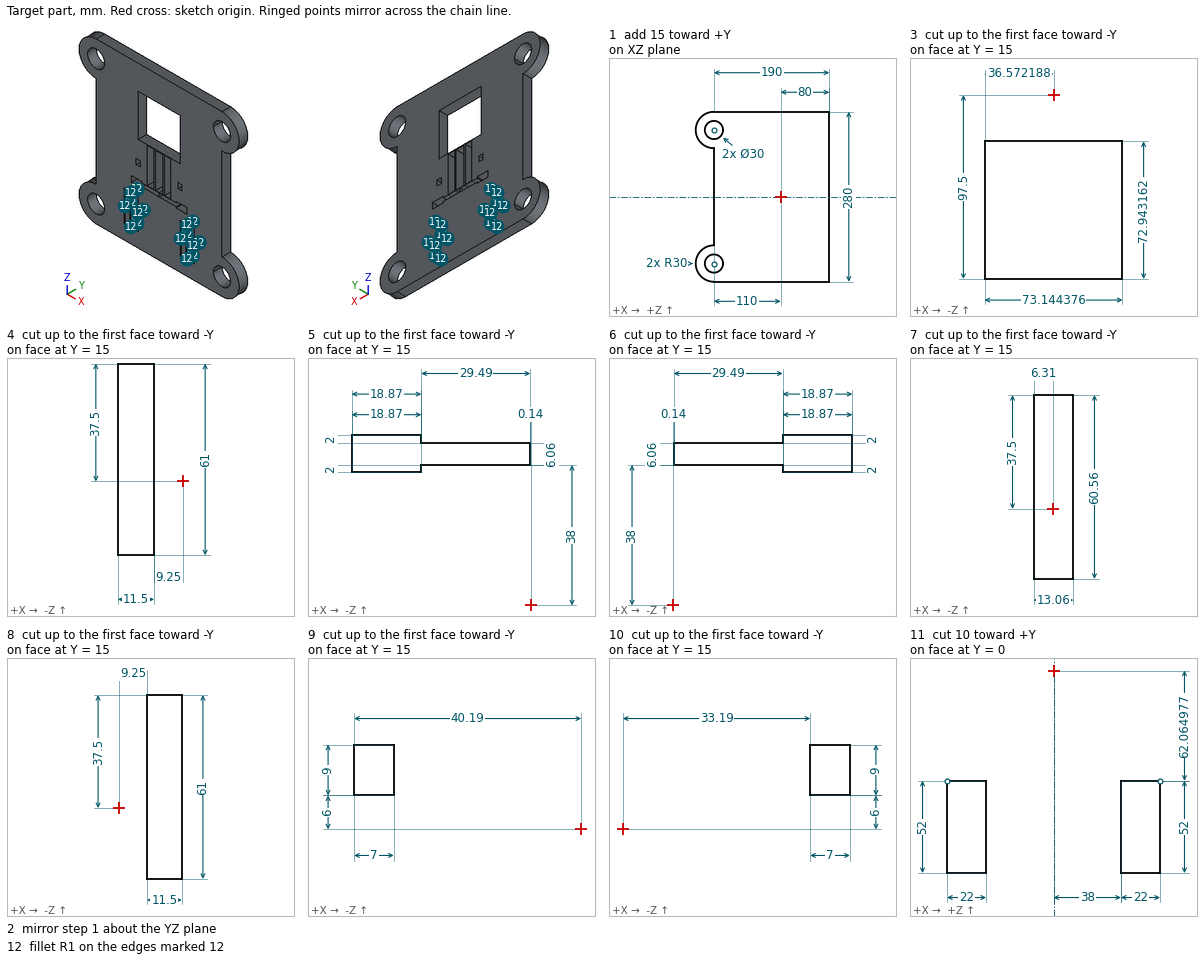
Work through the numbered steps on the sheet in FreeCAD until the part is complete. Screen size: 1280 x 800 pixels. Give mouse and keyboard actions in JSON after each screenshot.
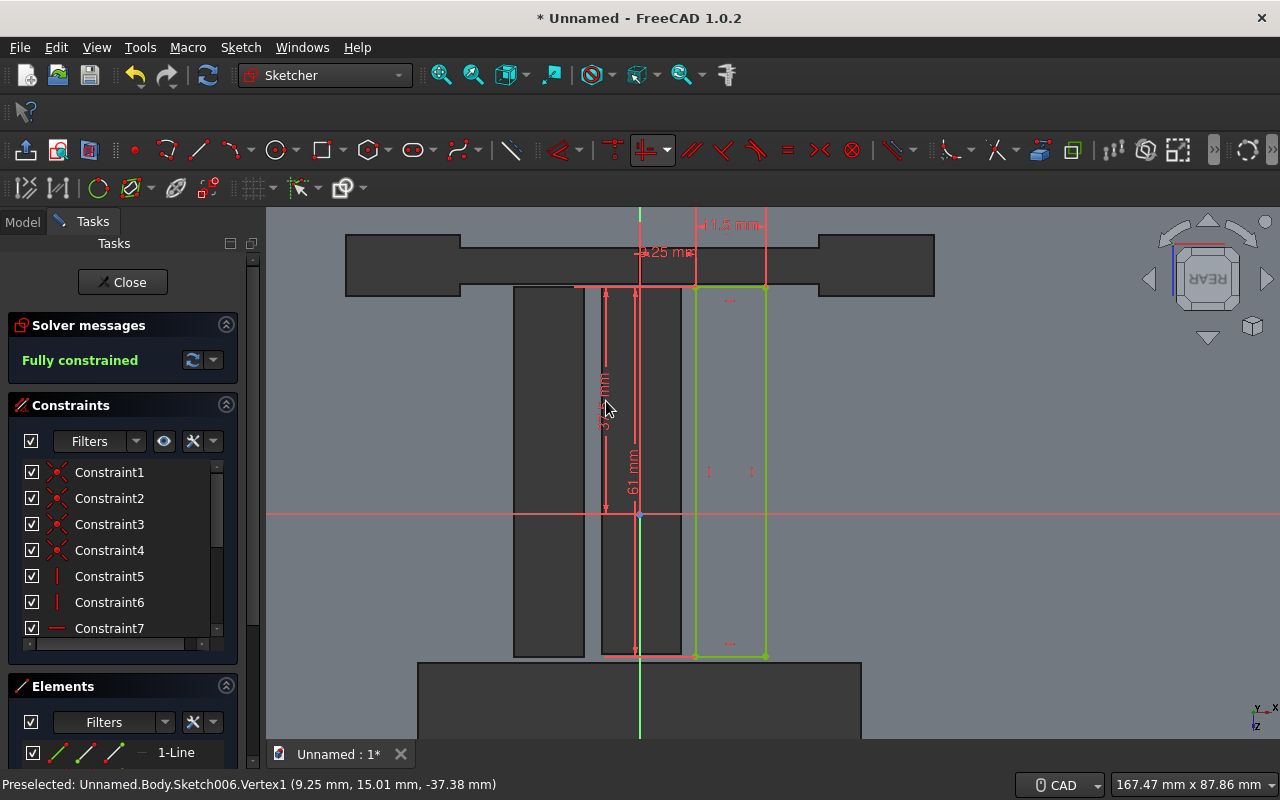
{"action": "left_click", "coordinate": [123, 282]}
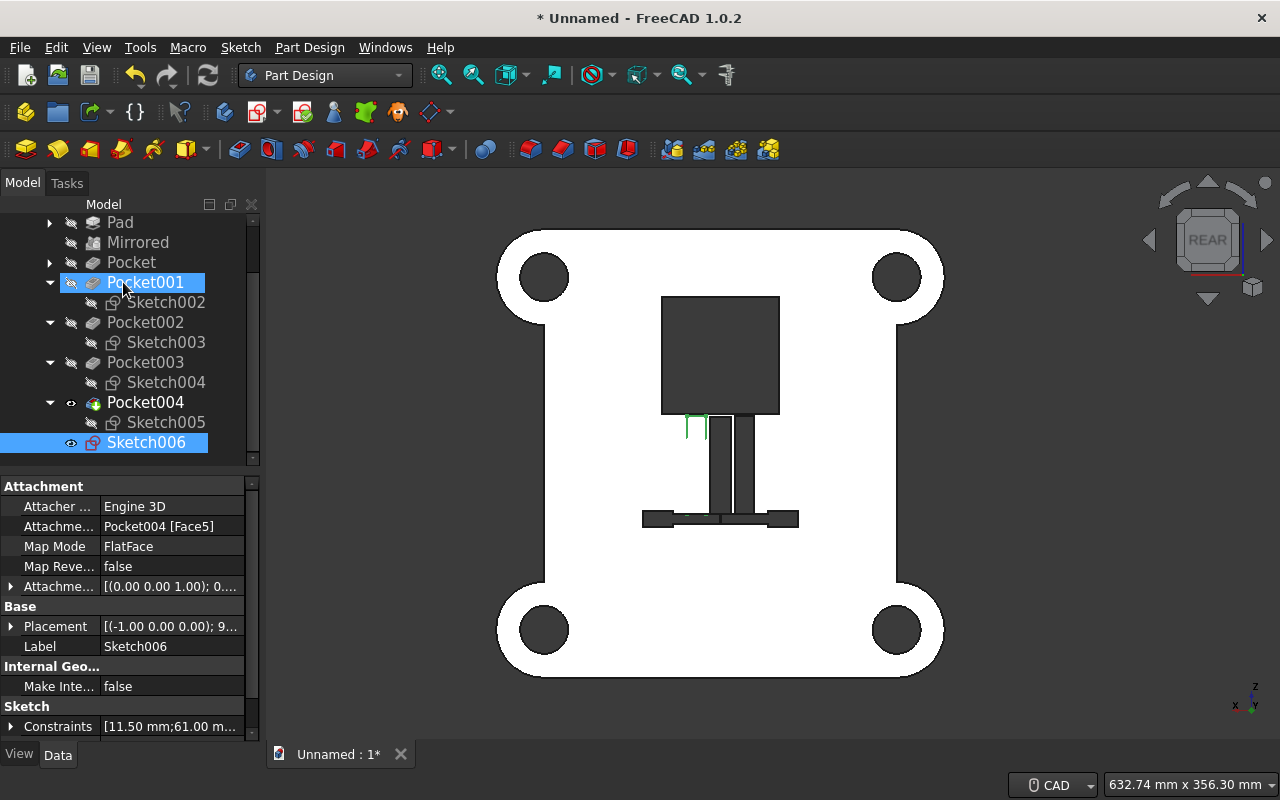
{"action": "left_click", "coordinate": [240, 150]}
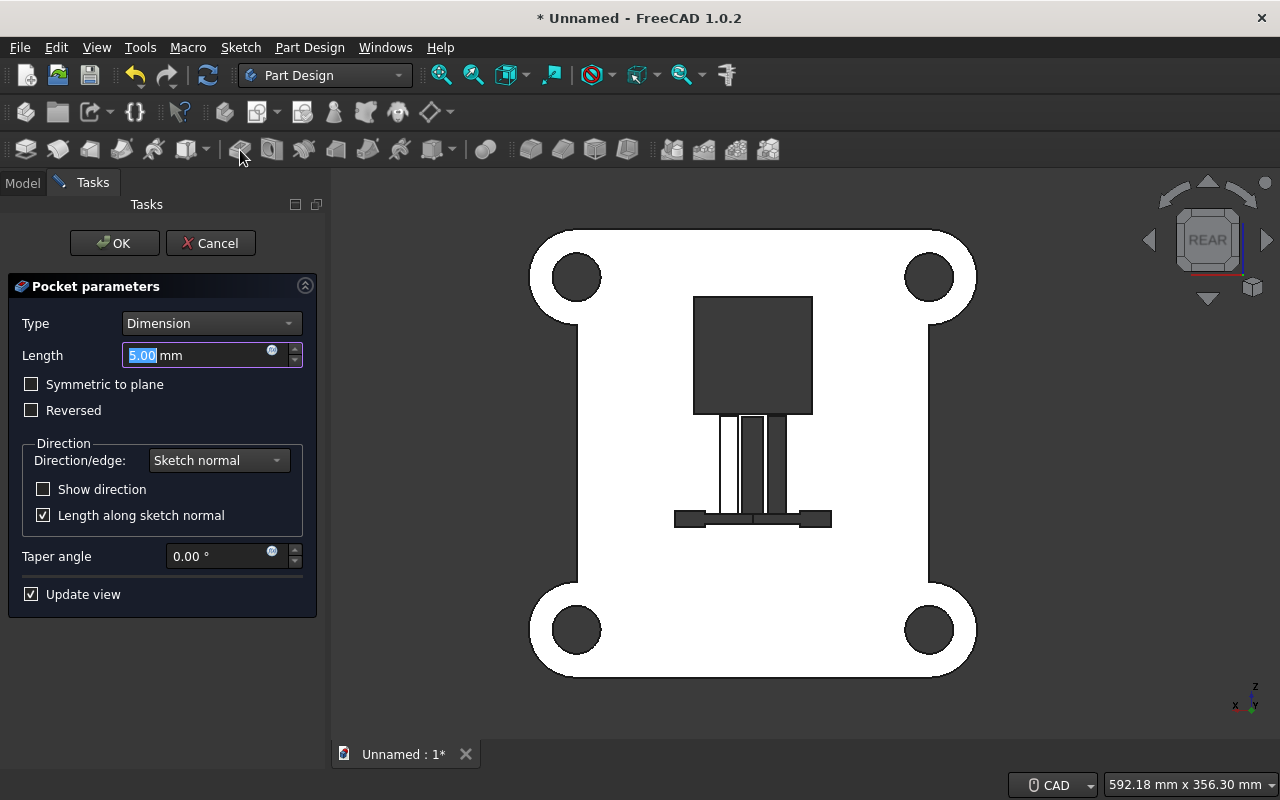
{"action": "left_click", "coordinate": [212, 324]}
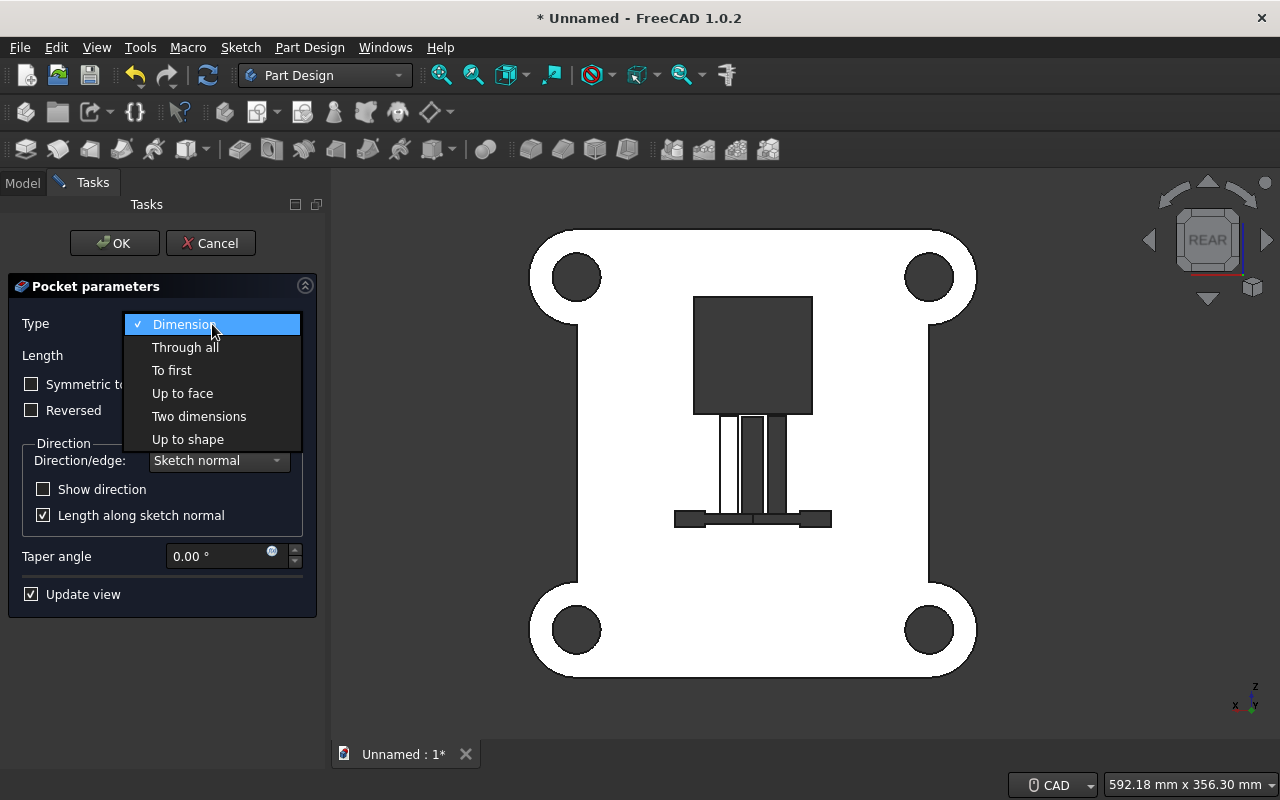
{"action": "left_click", "coordinate": [212, 370]}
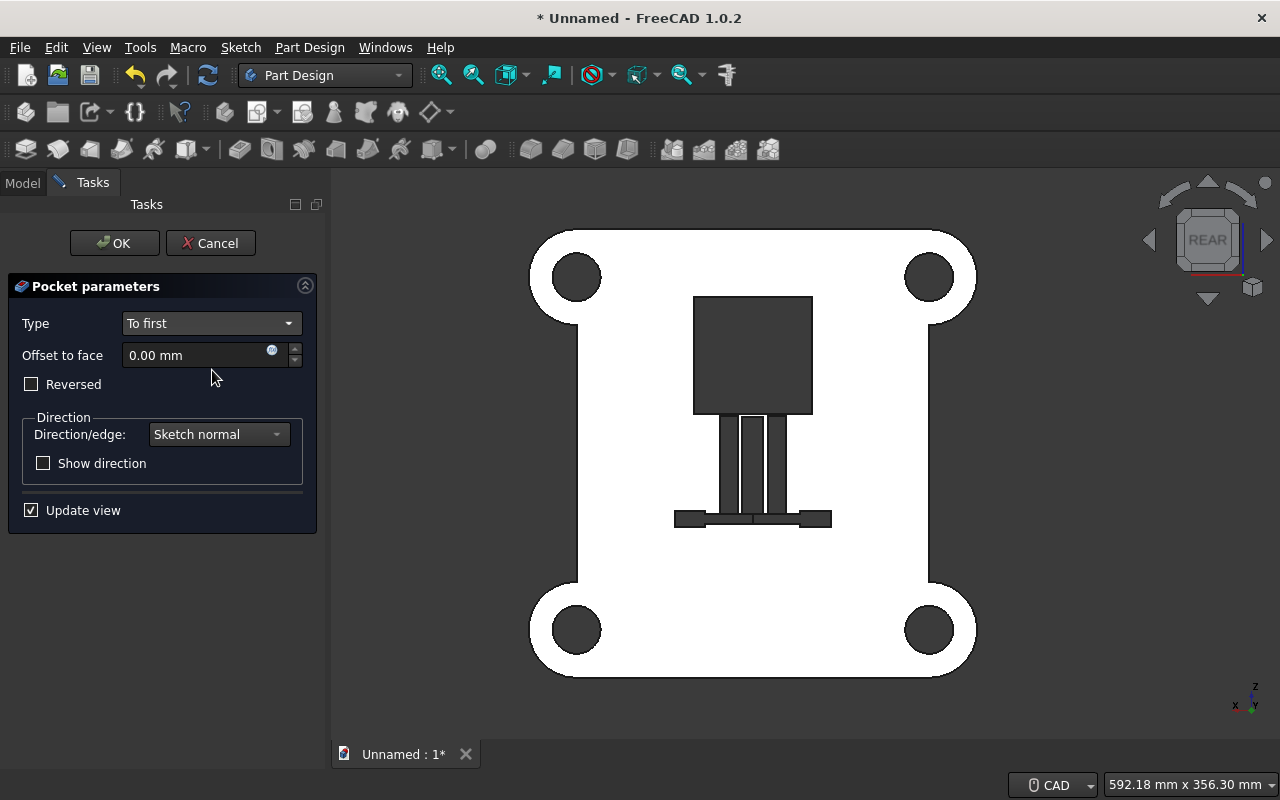
{"action": "left_click", "coordinate": [115, 243]}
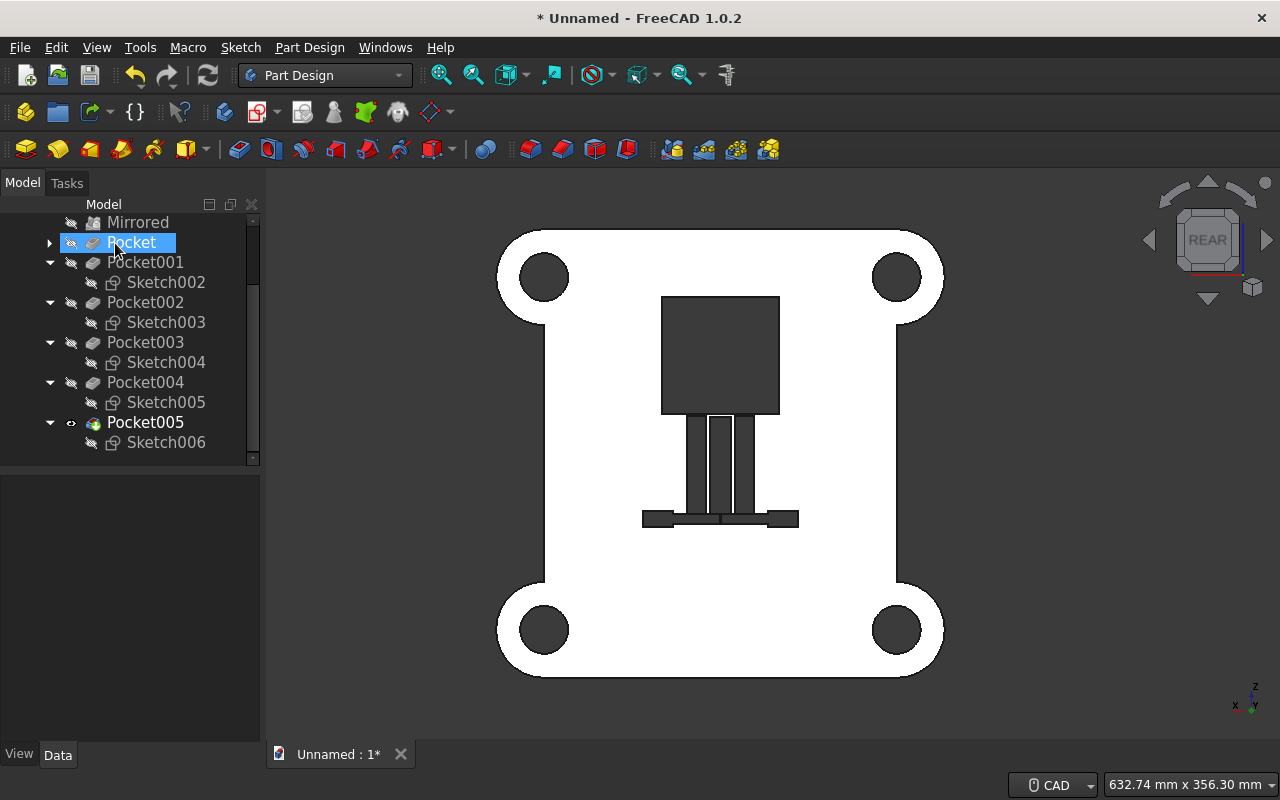
{"action": "left_click", "coordinate": [720, 581]}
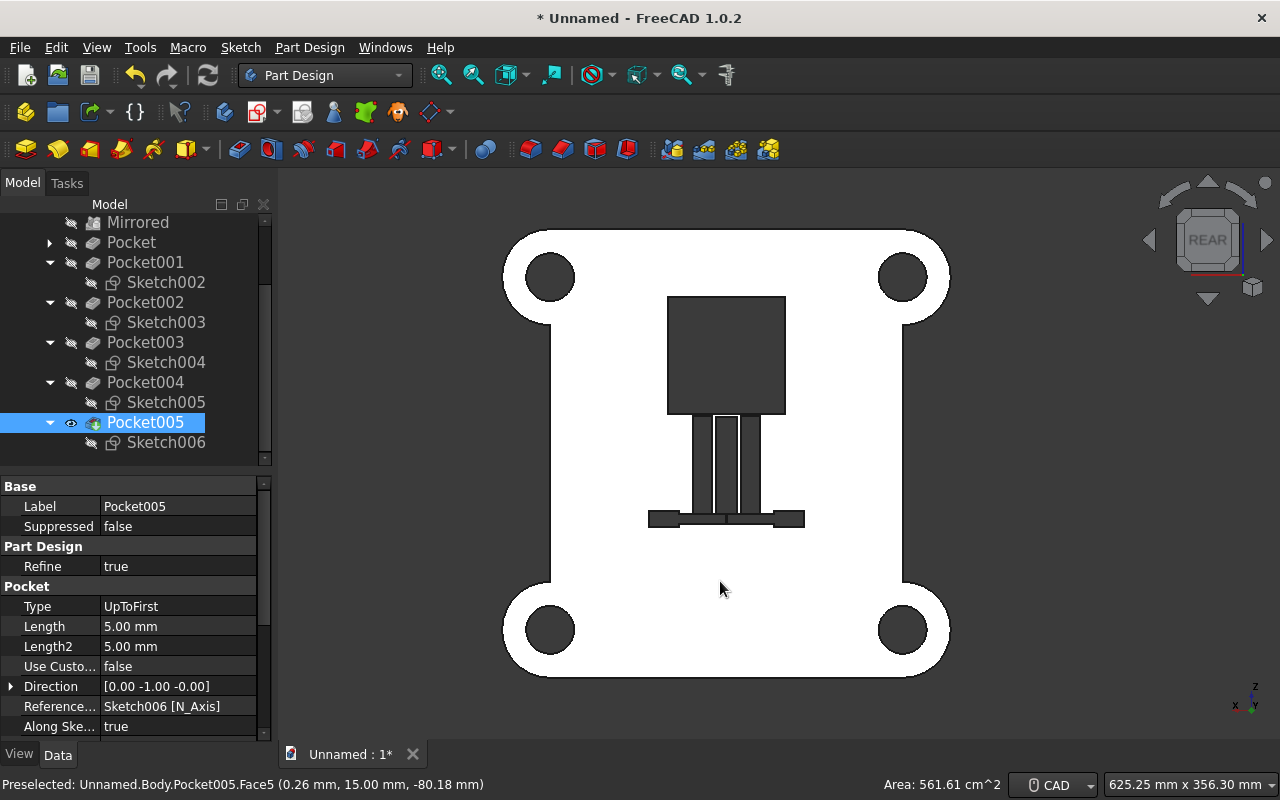
{"action": "left_click", "coordinate": [258, 112]}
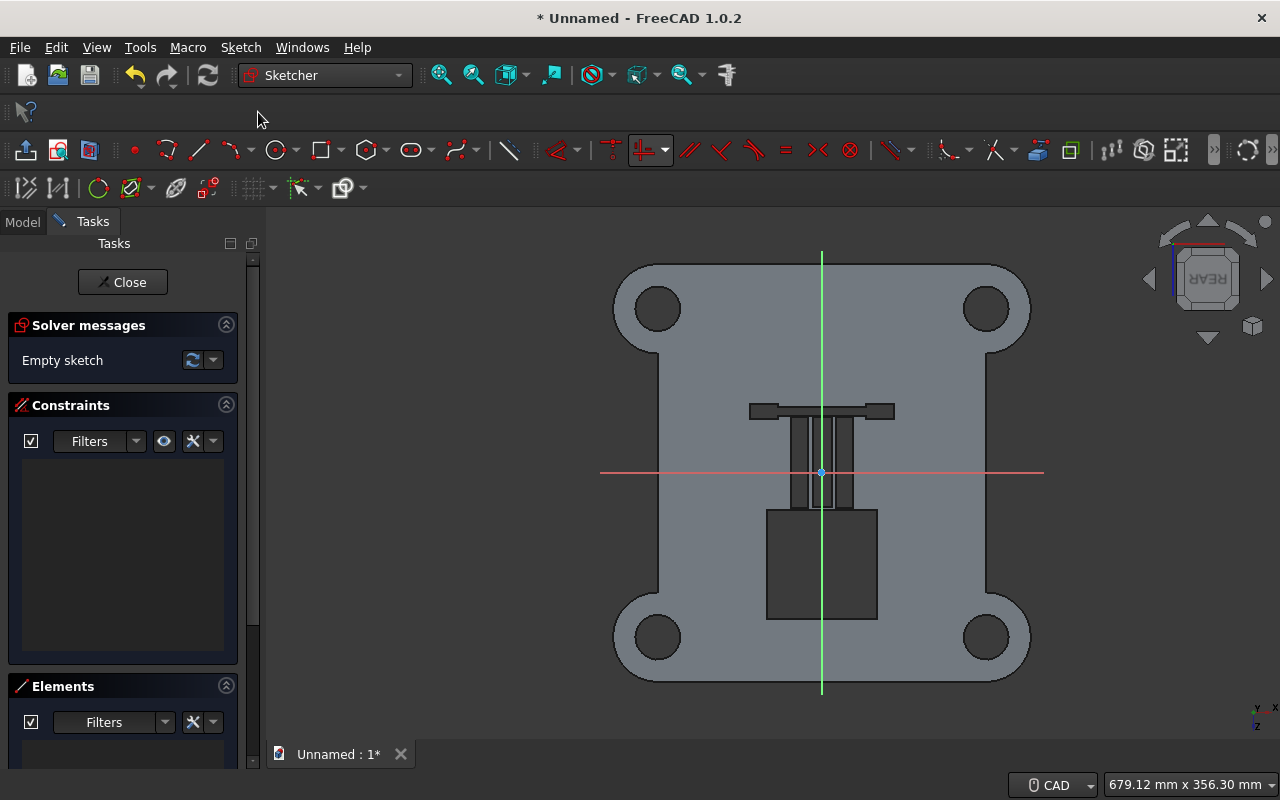
{"action": "scroll", "coordinate": [770, 457], "scroll_direction": "up", "scroll_amount": 15}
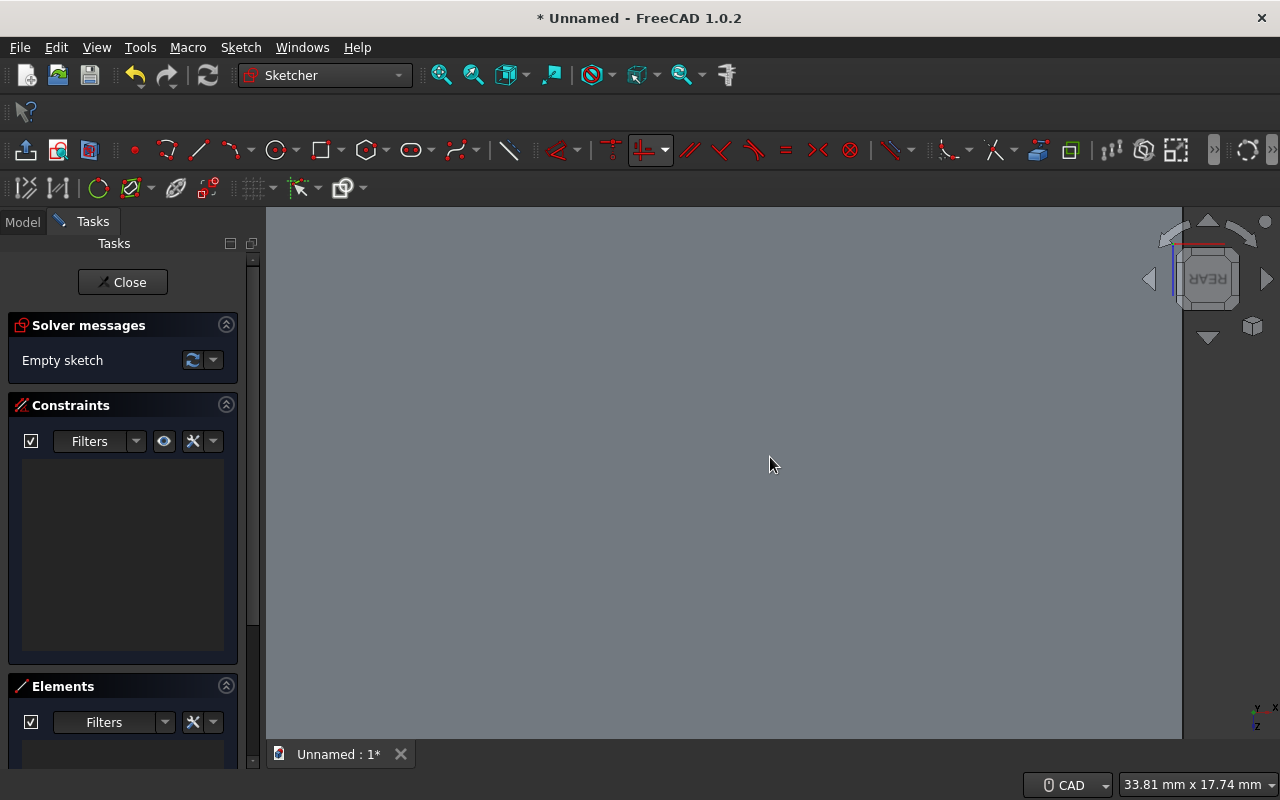
{"action": "left_click", "coordinate": [322, 150]}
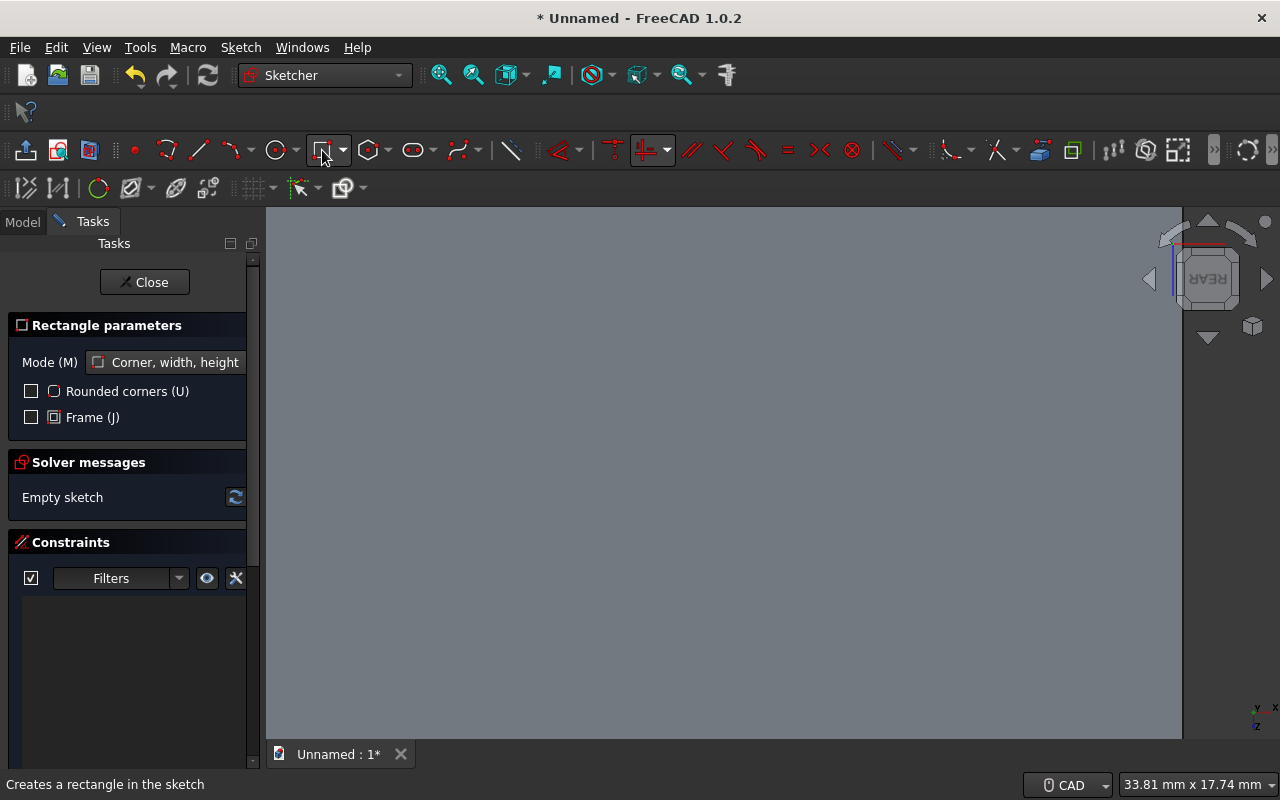
{"action": "left_click", "coordinate": [600, 320]}
{"action": "mouse_move", "coordinate": [809, 589]}